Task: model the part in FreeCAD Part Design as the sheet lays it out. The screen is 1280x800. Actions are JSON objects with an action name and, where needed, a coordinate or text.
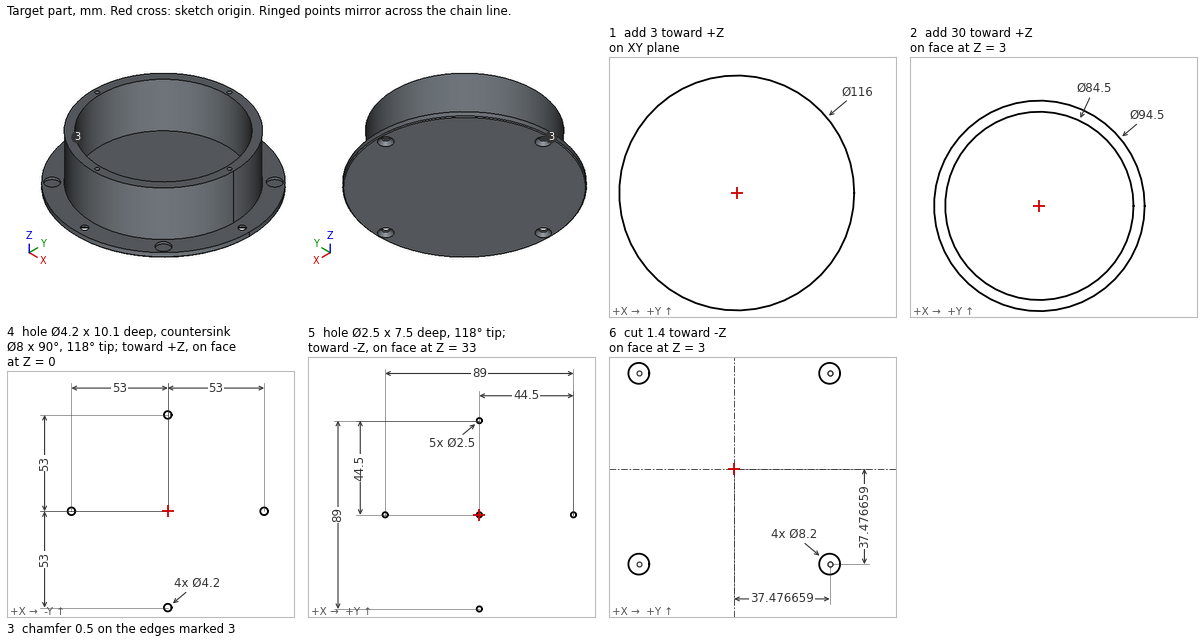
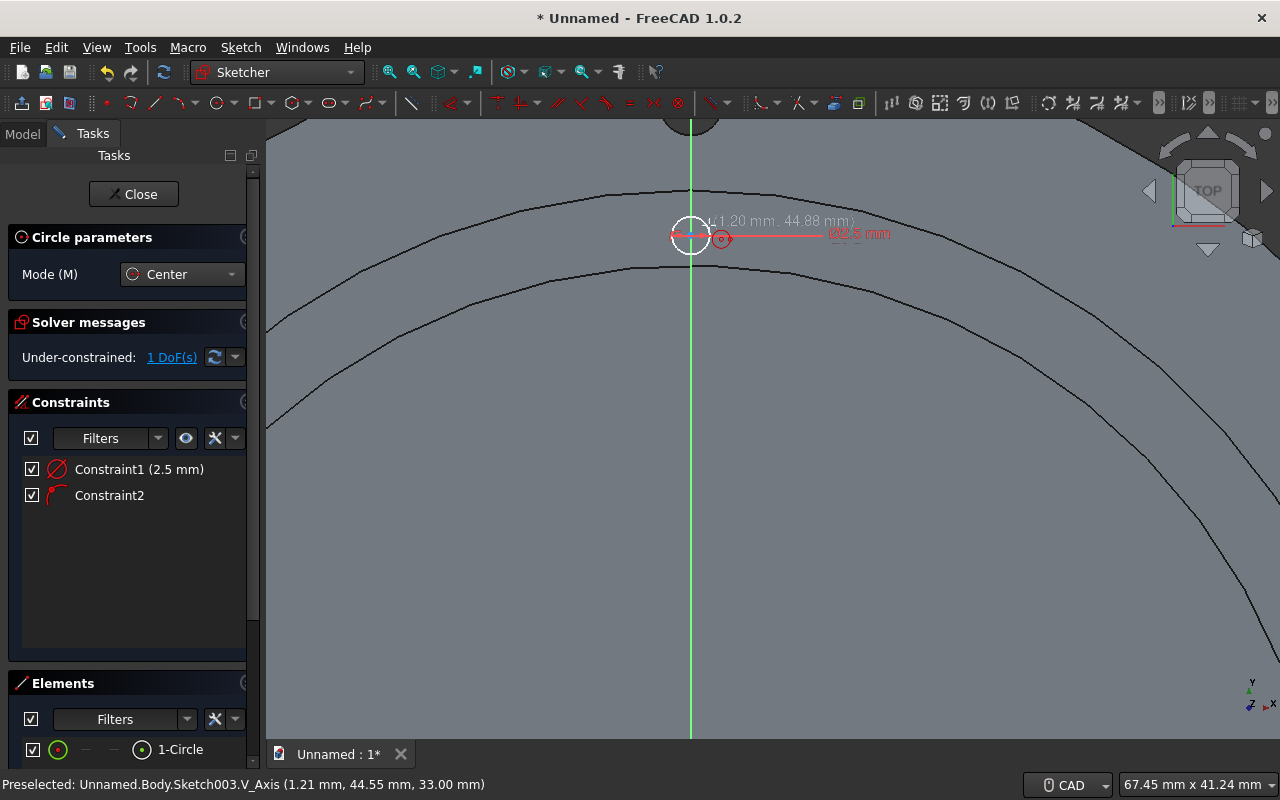
{"action": "scroll", "coordinate": [710, 226], "scroll_direction": "down", "scroll_amount": 6}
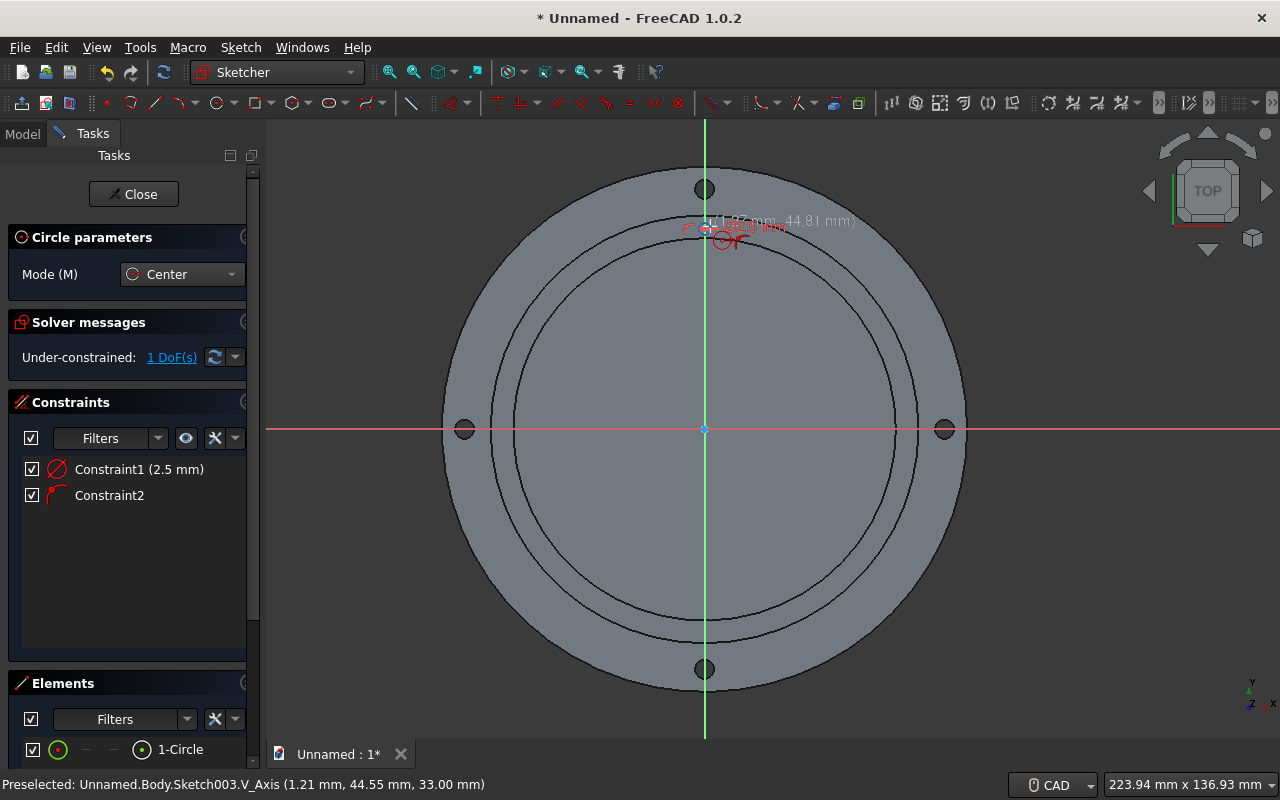
{"action": "scroll", "coordinate": [906, 429], "scroll_direction": "up", "scroll_amount": 7}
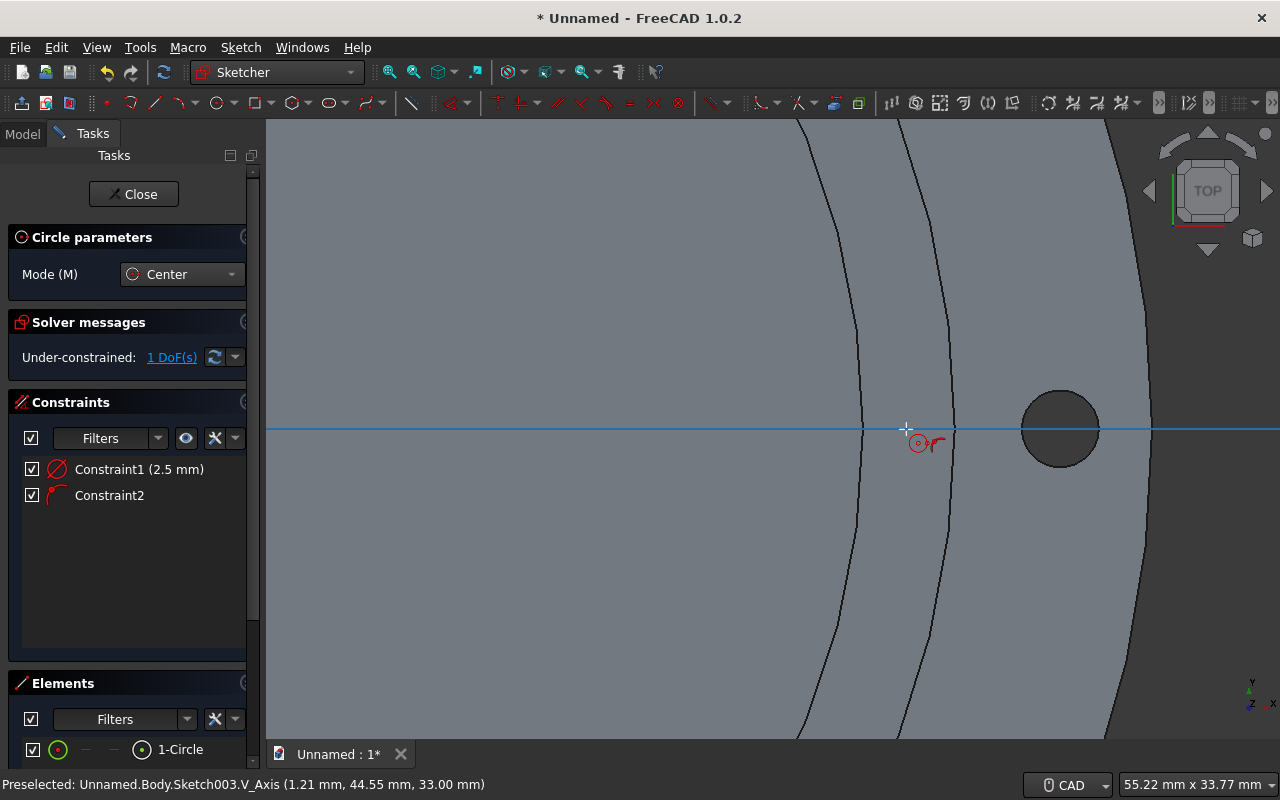
{"action": "scroll", "coordinate": [907, 429], "scroll_direction": "down", "scroll_amount": 7}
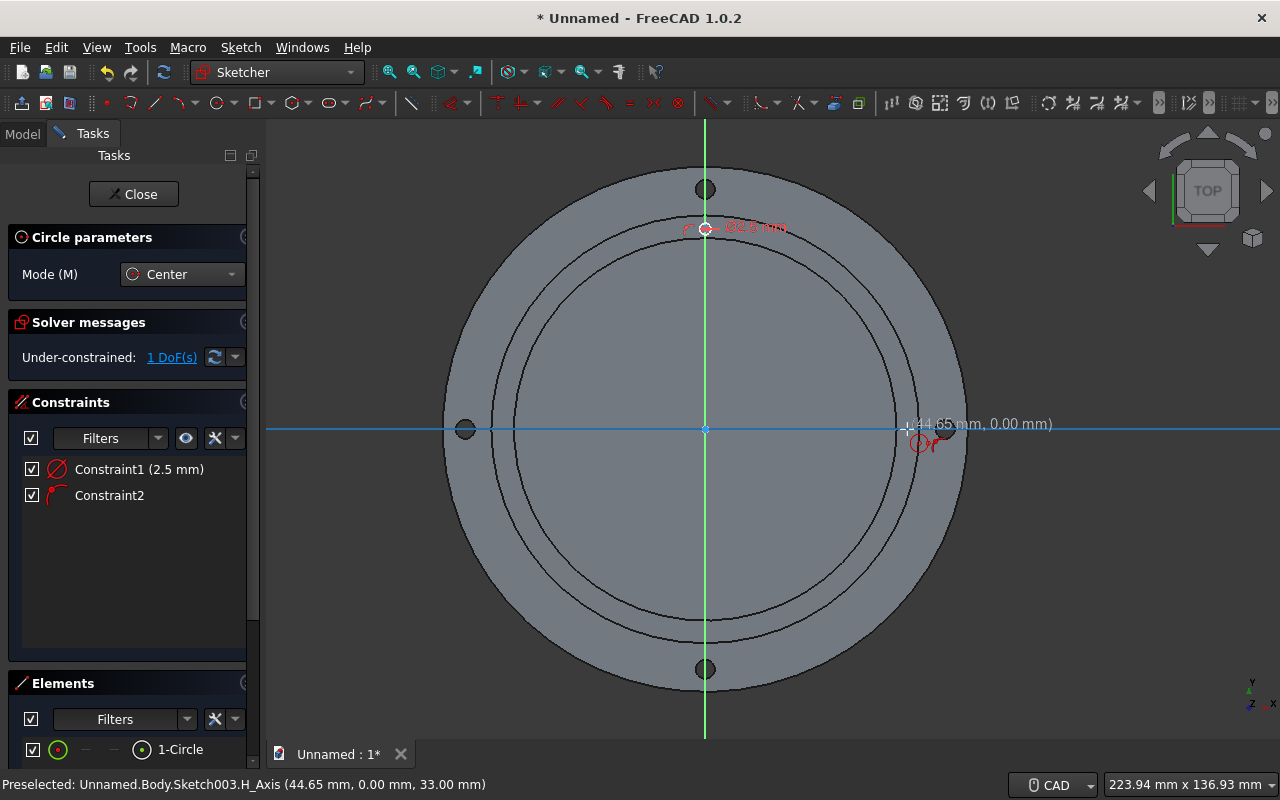
{"action": "left_click", "coordinate": [907, 429]}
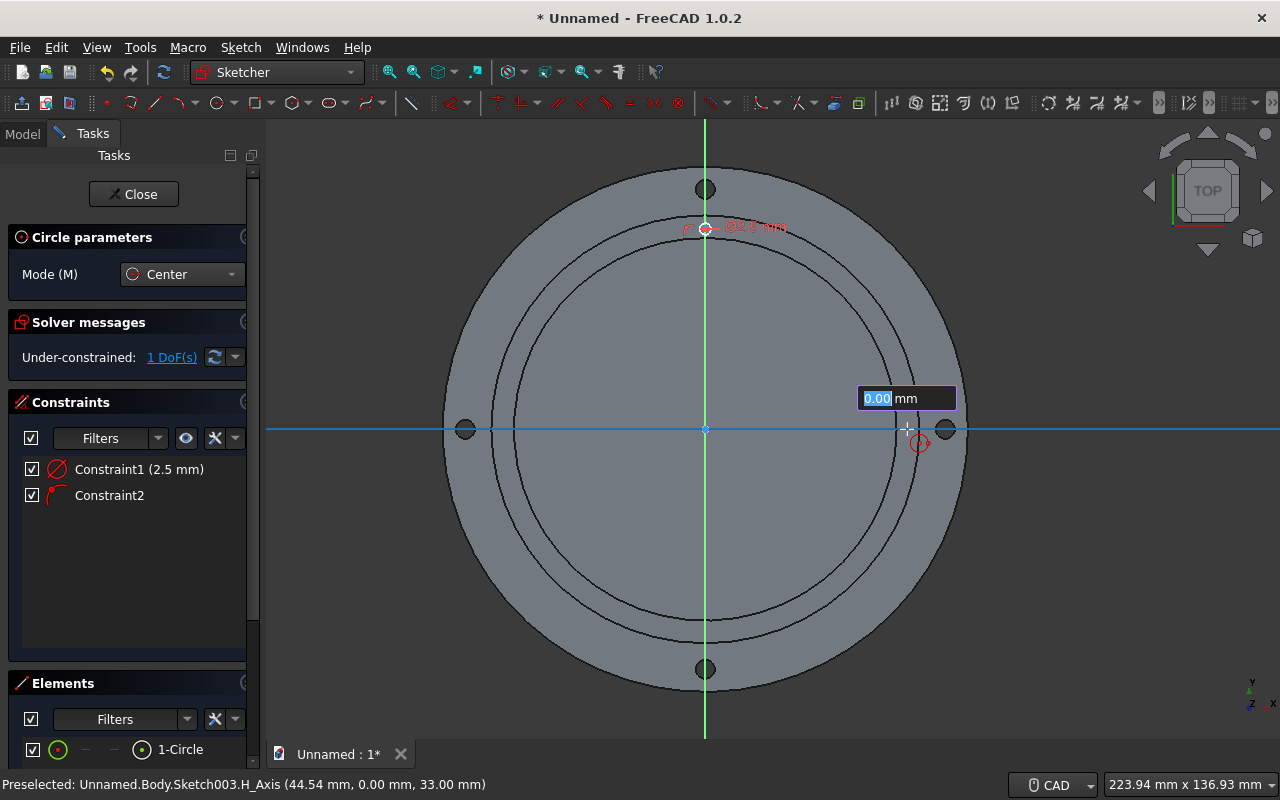
{"action": "scroll", "coordinate": [905, 435], "scroll_direction": "up", "scroll_amount": 6}
{"action": "mouse_move", "coordinate": [903, 433]}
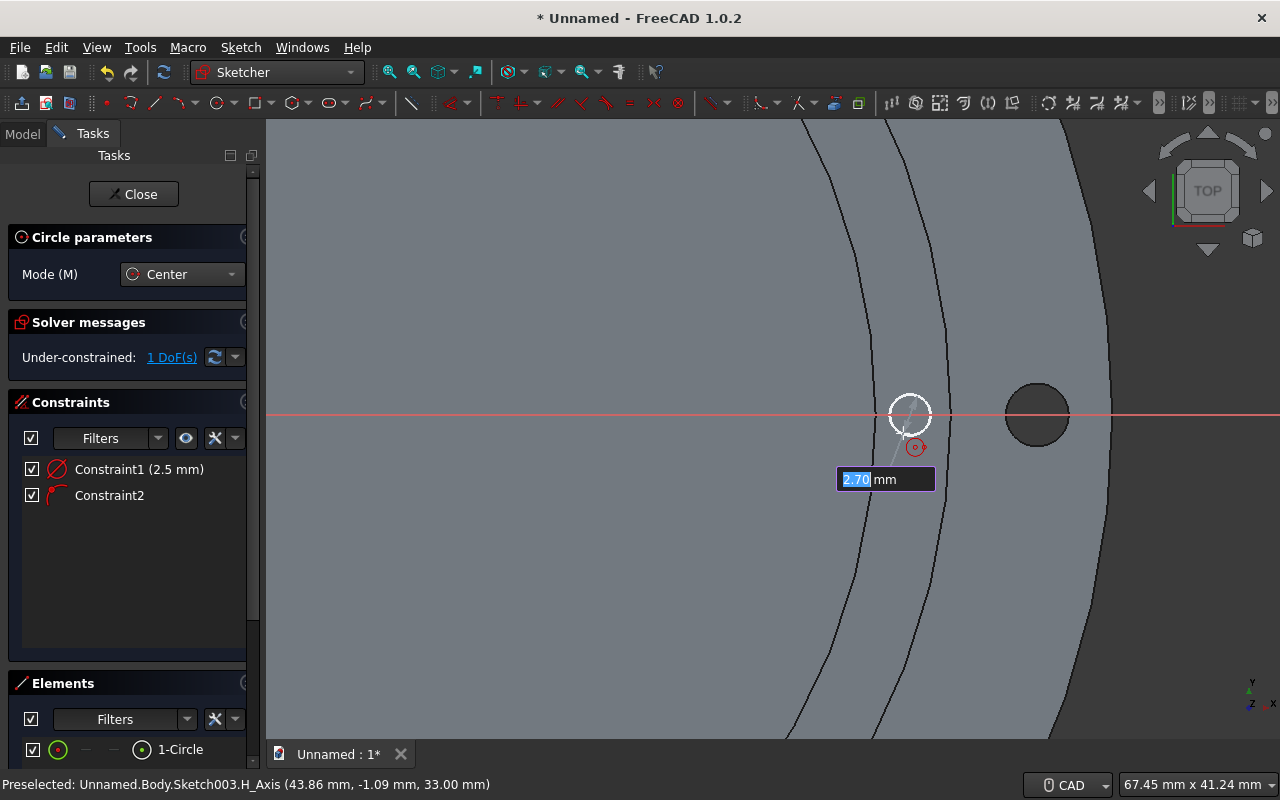
{"action": "type", "text": "2.5"}
{"action": "key", "text": "Return"}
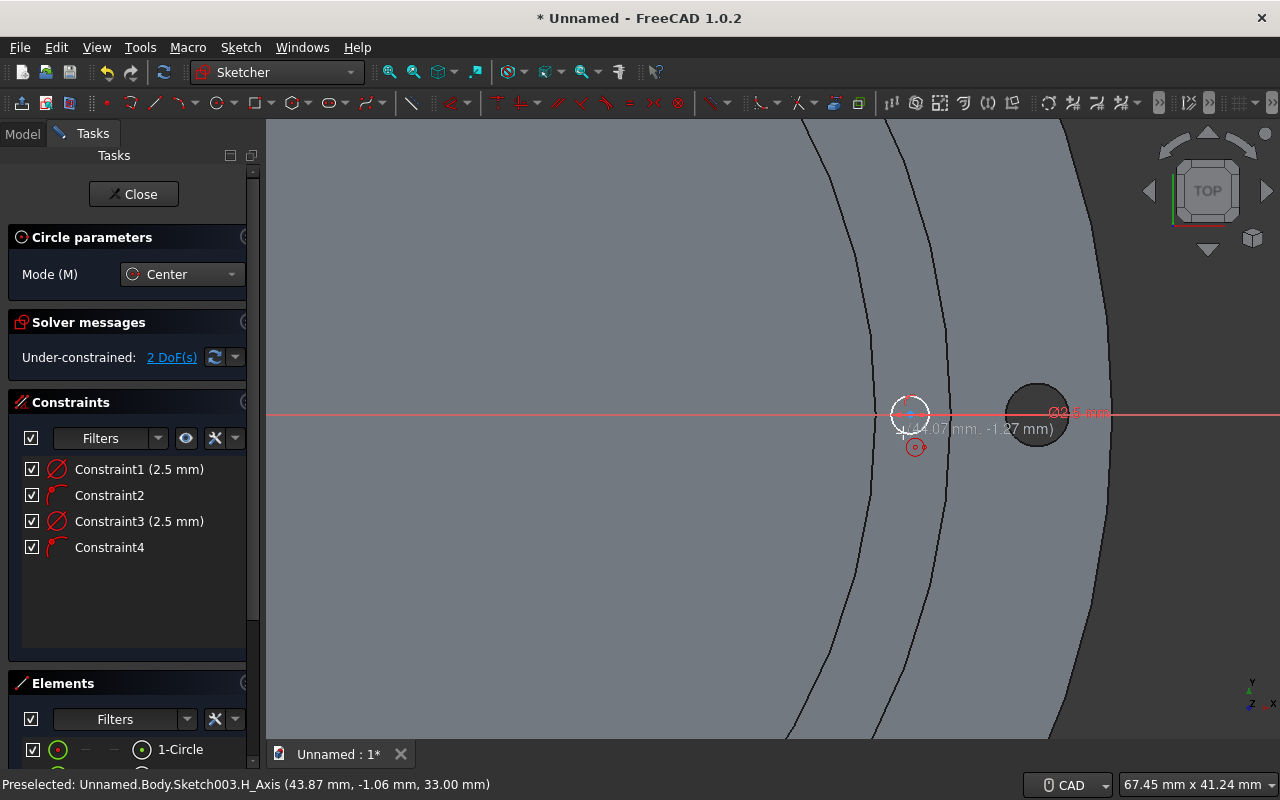
{"action": "scroll", "coordinate": [904, 435], "scroll_direction": "down", "scroll_amount": 6}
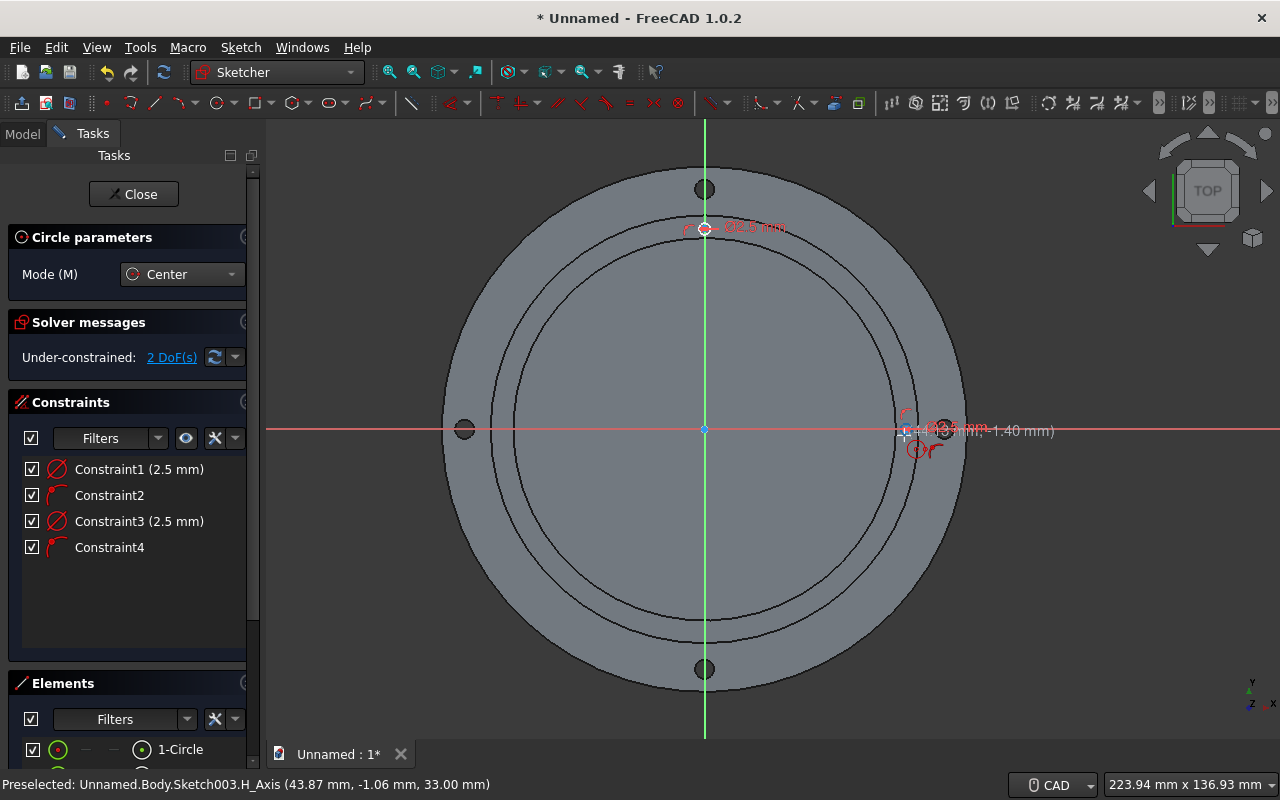
{"action": "scroll", "coordinate": [705, 631], "scroll_direction": "up", "scroll_amount": 7}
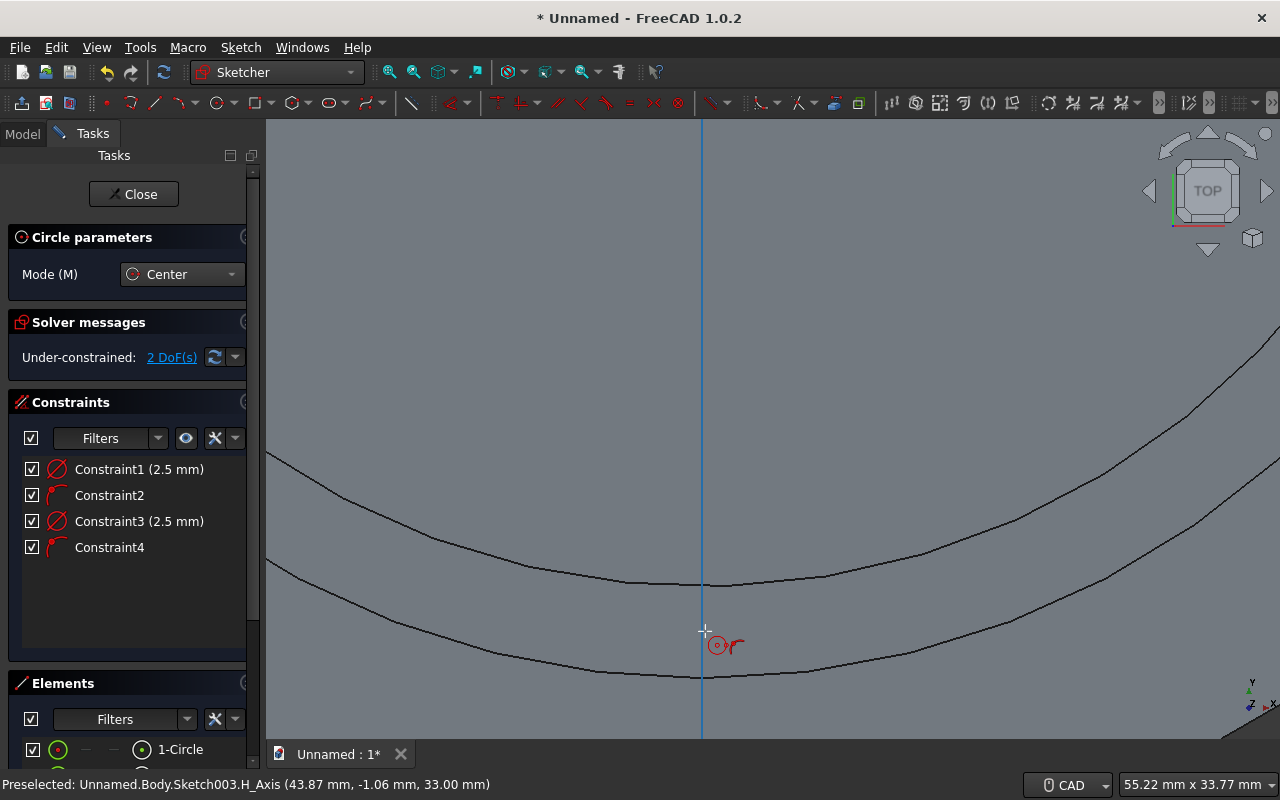
{"action": "scroll", "coordinate": [705, 631], "scroll_direction": "down", "scroll_amount": 7}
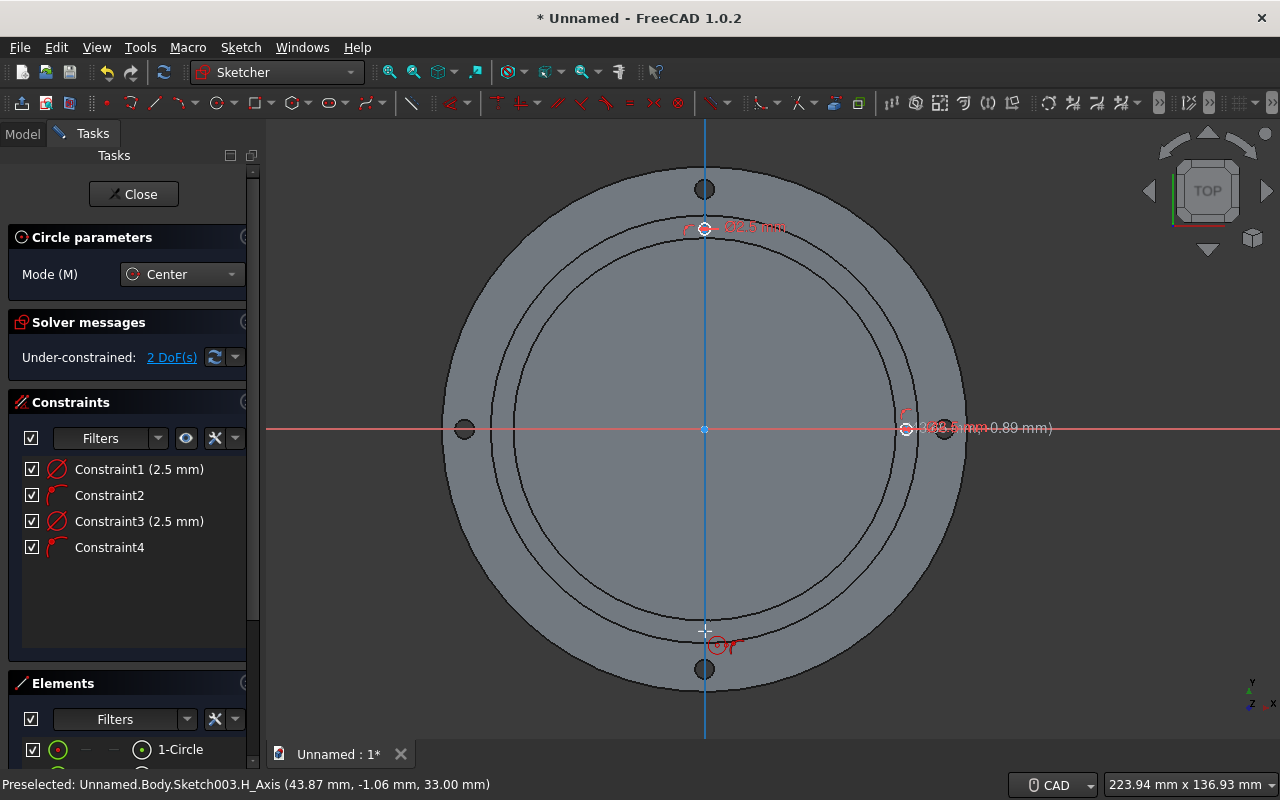
{"action": "left_click", "coordinate": [705, 631]}